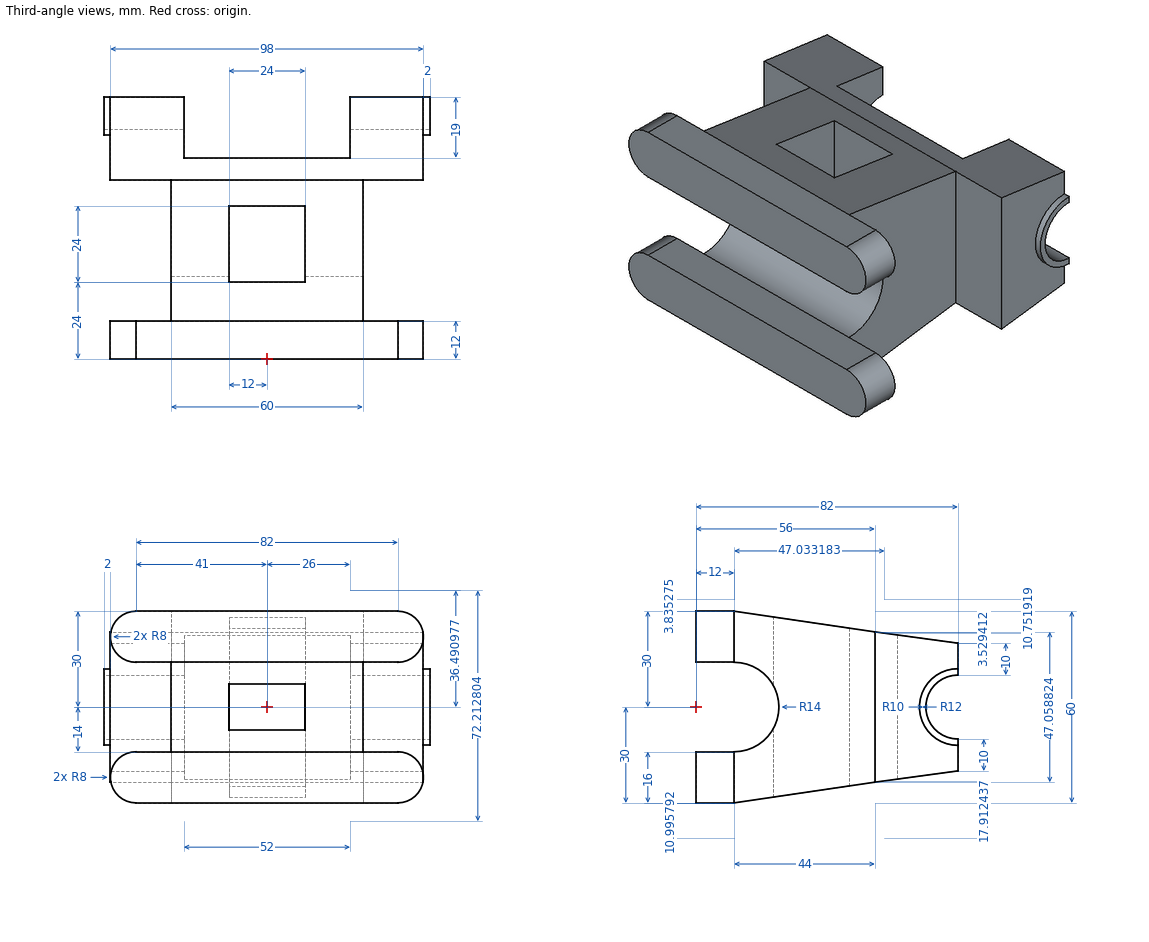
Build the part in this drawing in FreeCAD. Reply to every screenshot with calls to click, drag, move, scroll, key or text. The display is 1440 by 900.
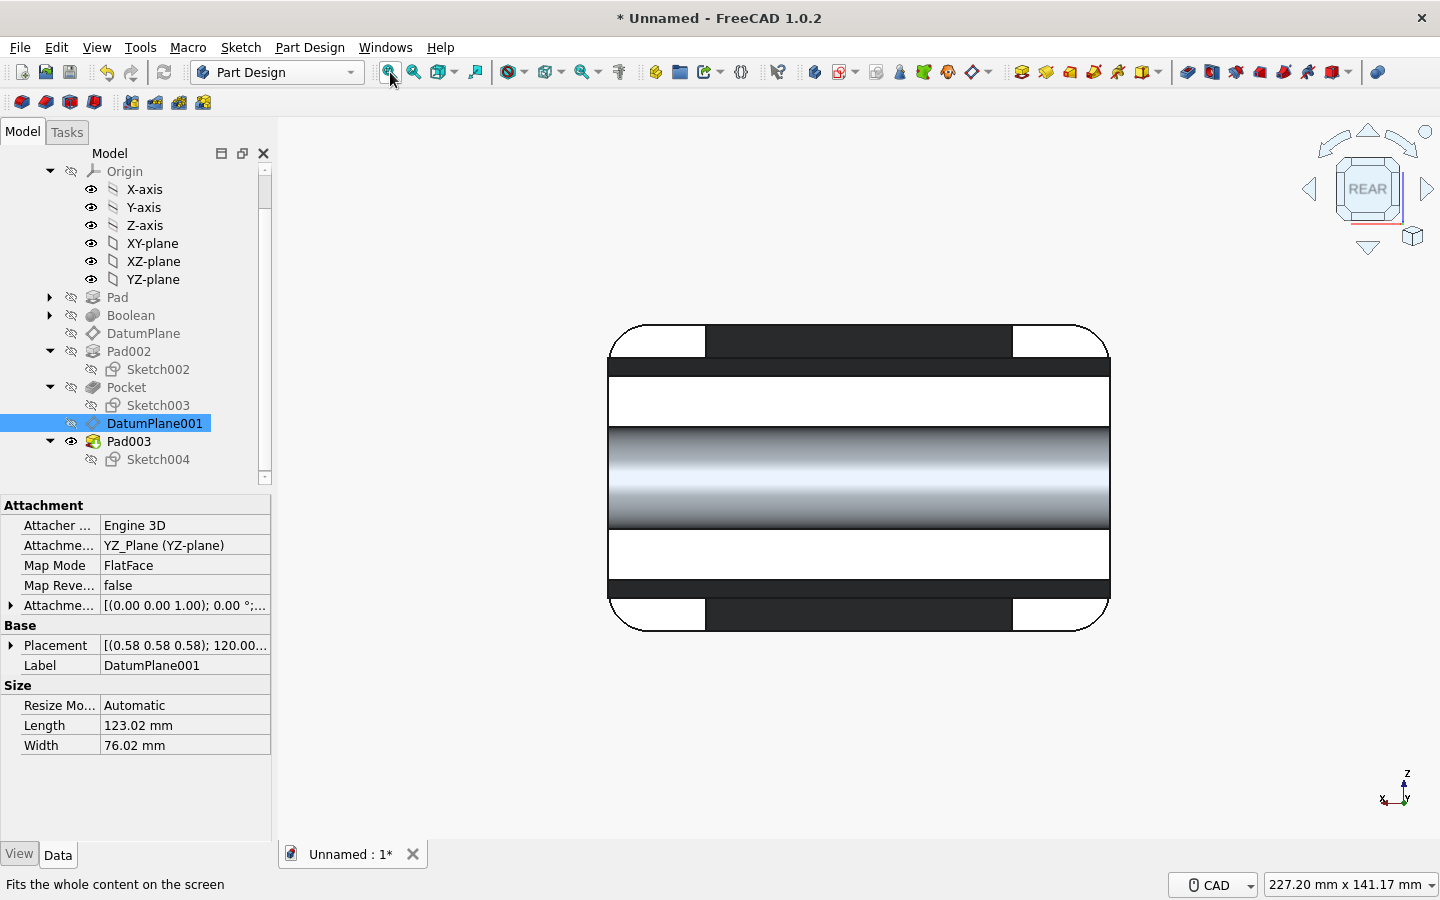
click(390, 72)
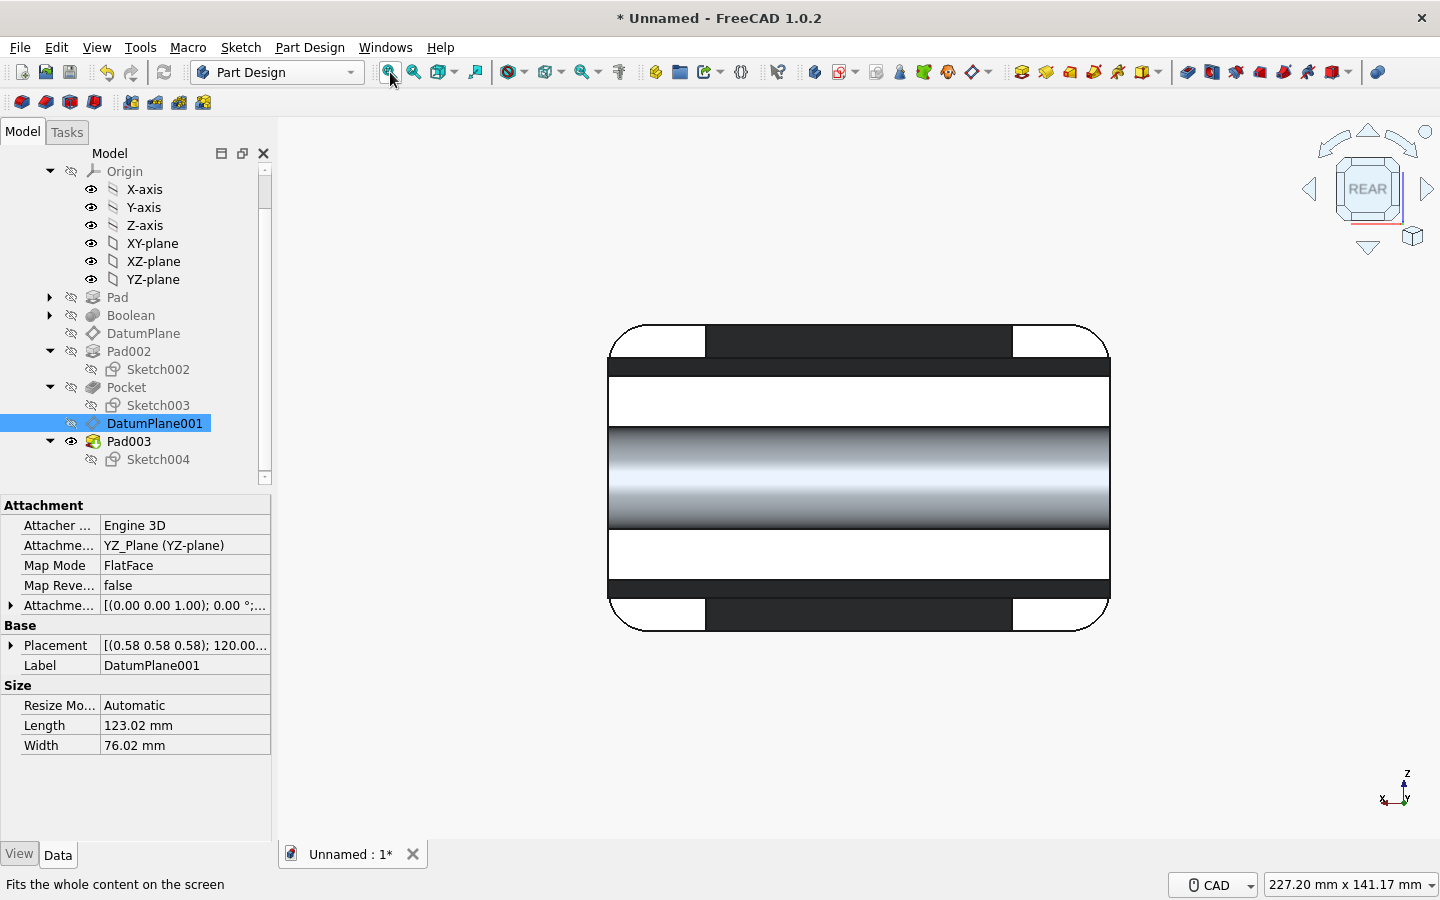
click(644, 554)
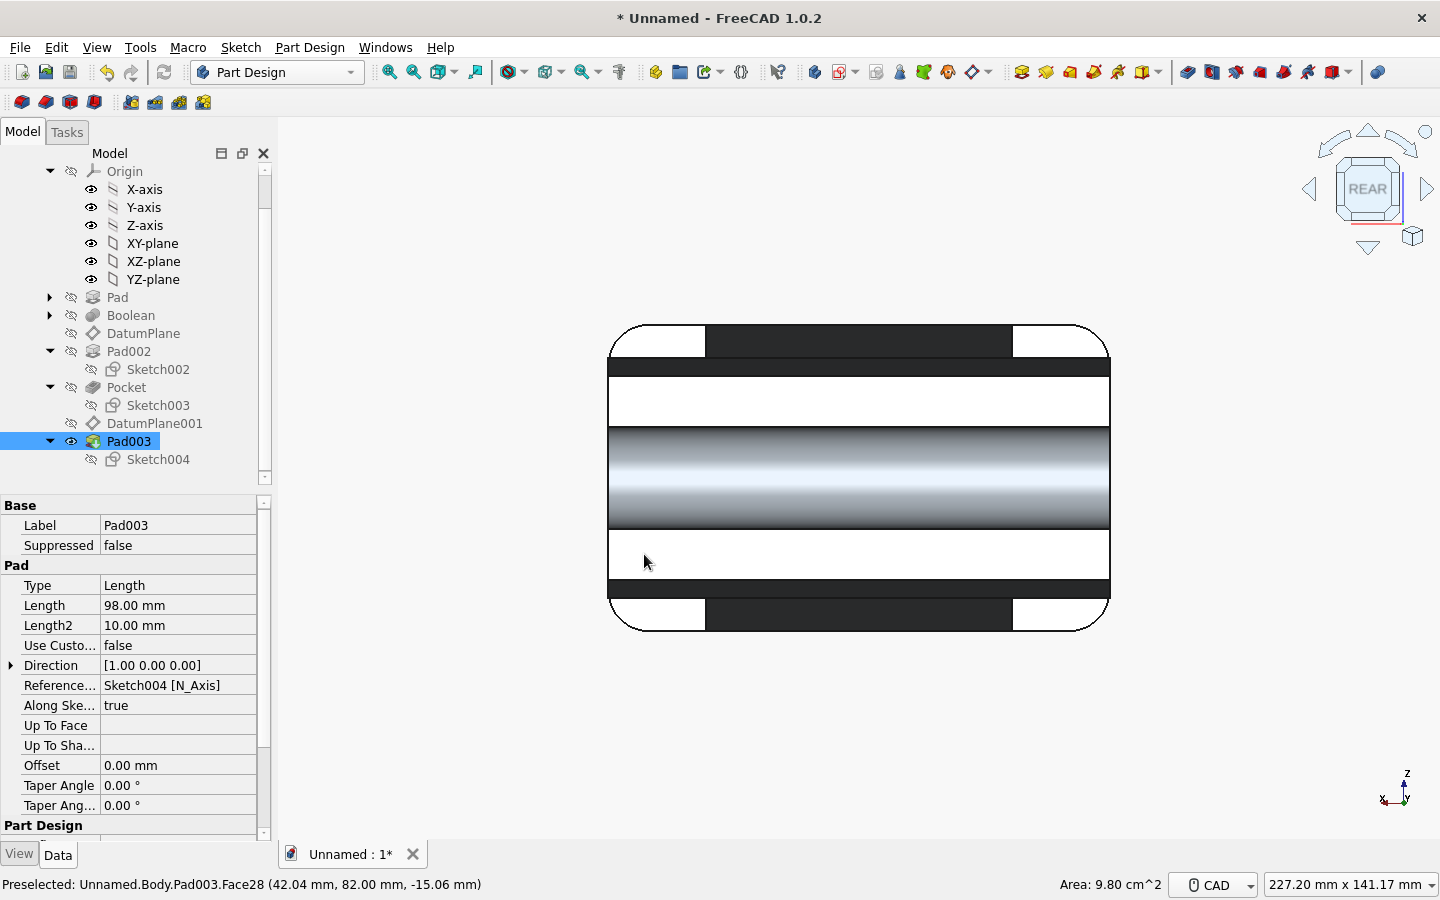
click(840, 72)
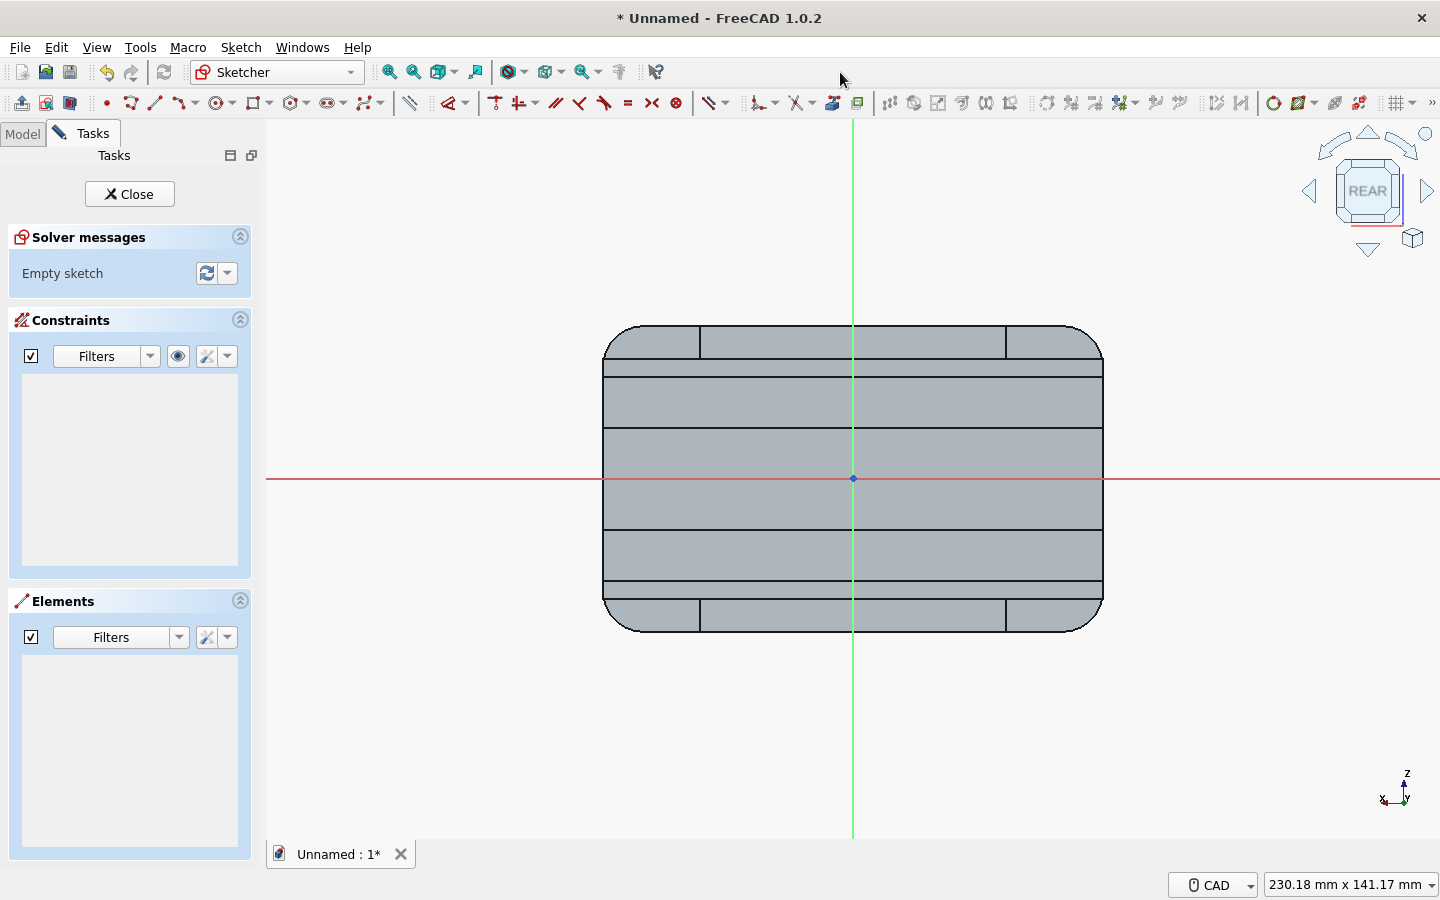
click(254, 104)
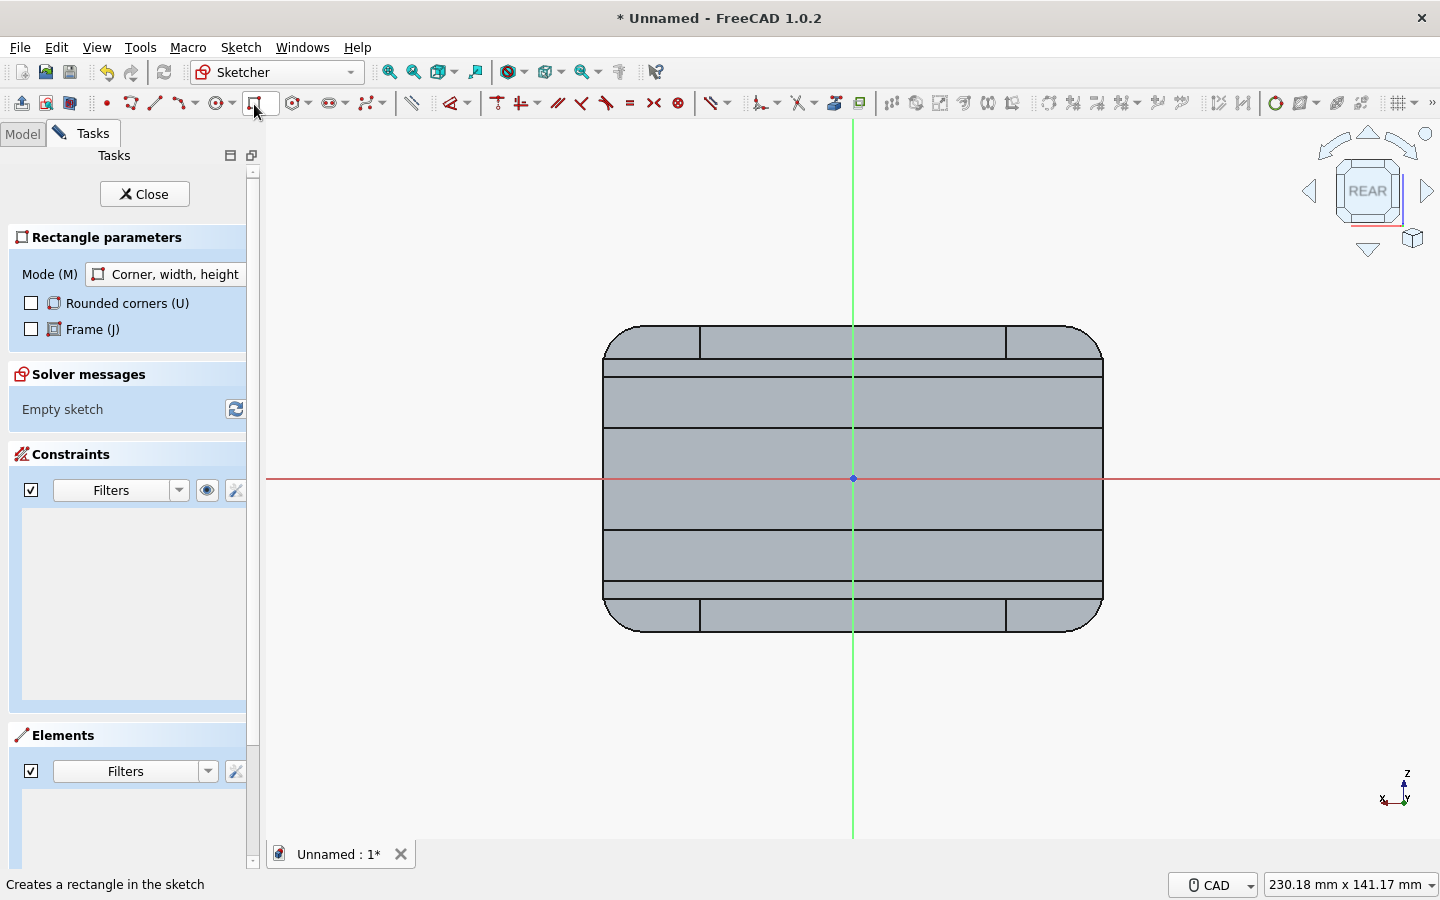
click(720, 293)
click(986, 661)
key(Escape)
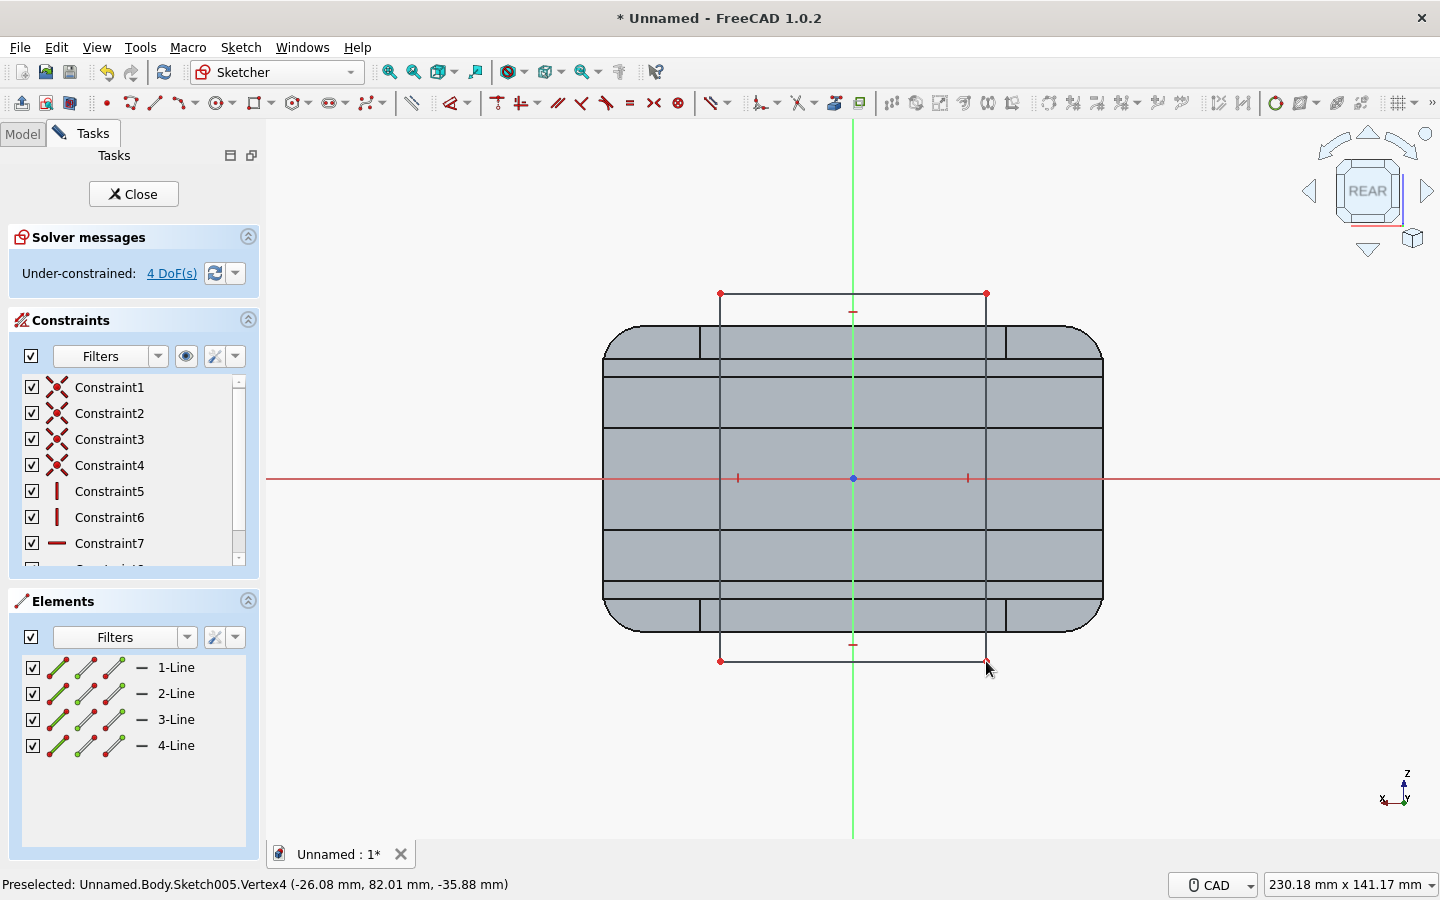
click(450, 104)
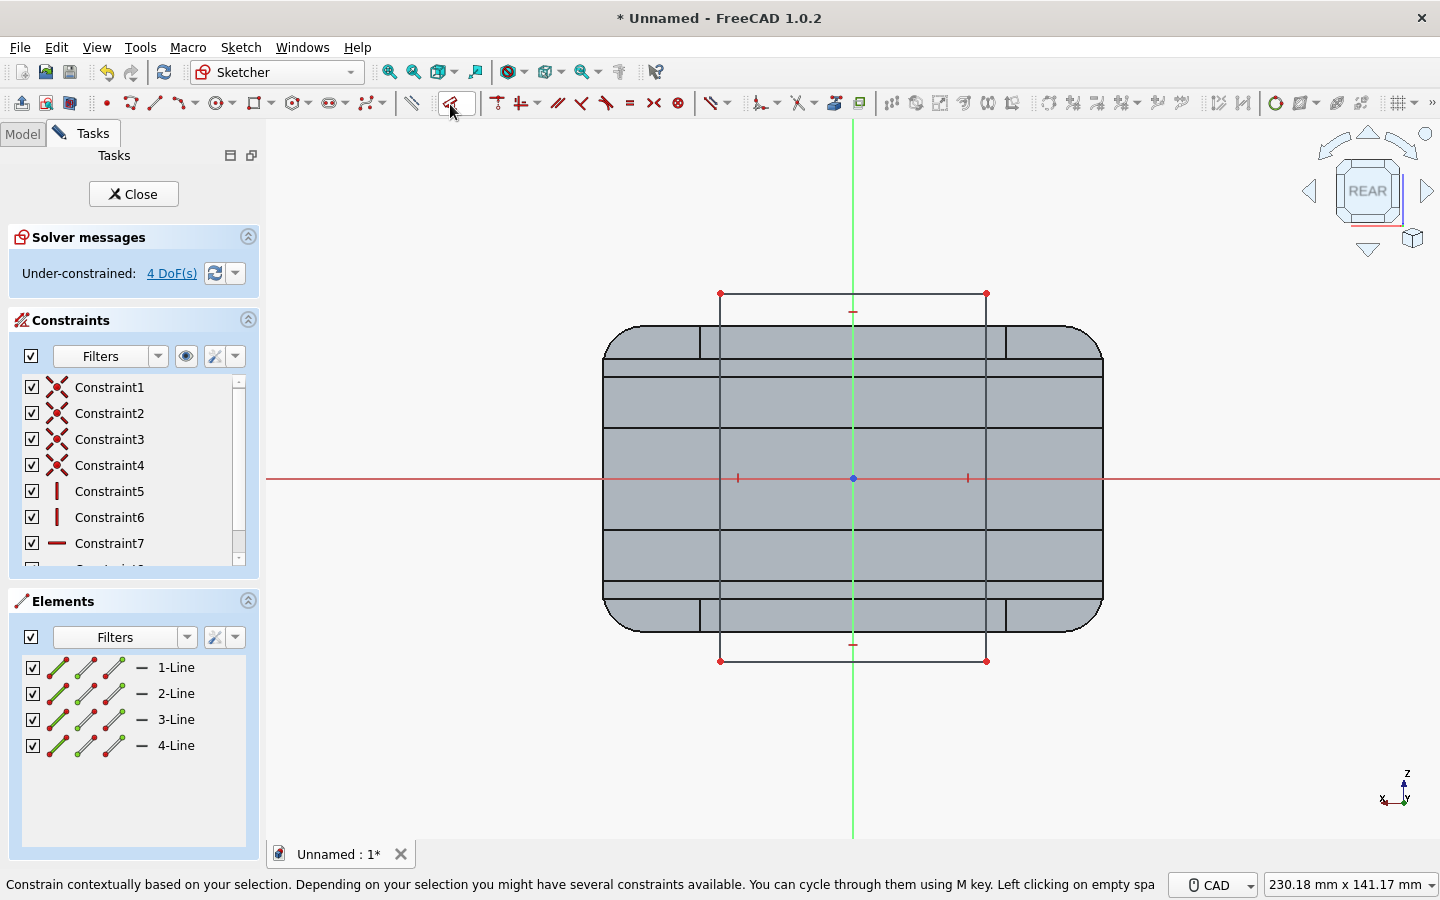
click(800, 662)
click(792, 696)